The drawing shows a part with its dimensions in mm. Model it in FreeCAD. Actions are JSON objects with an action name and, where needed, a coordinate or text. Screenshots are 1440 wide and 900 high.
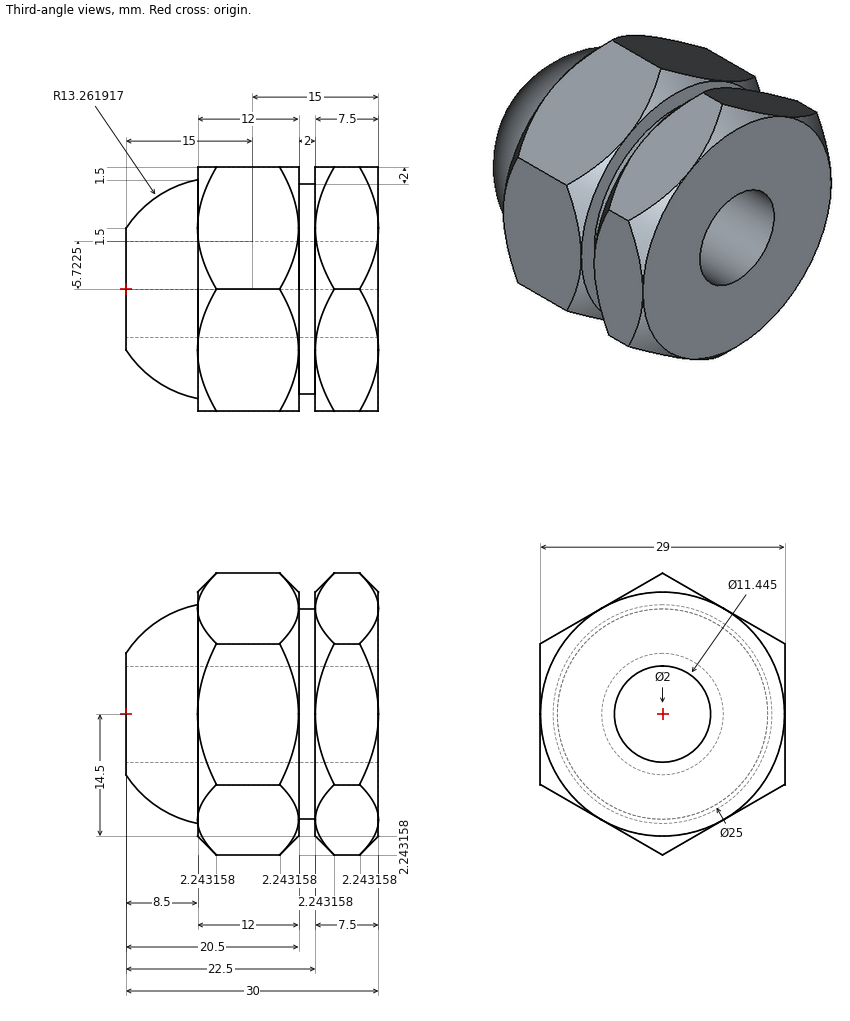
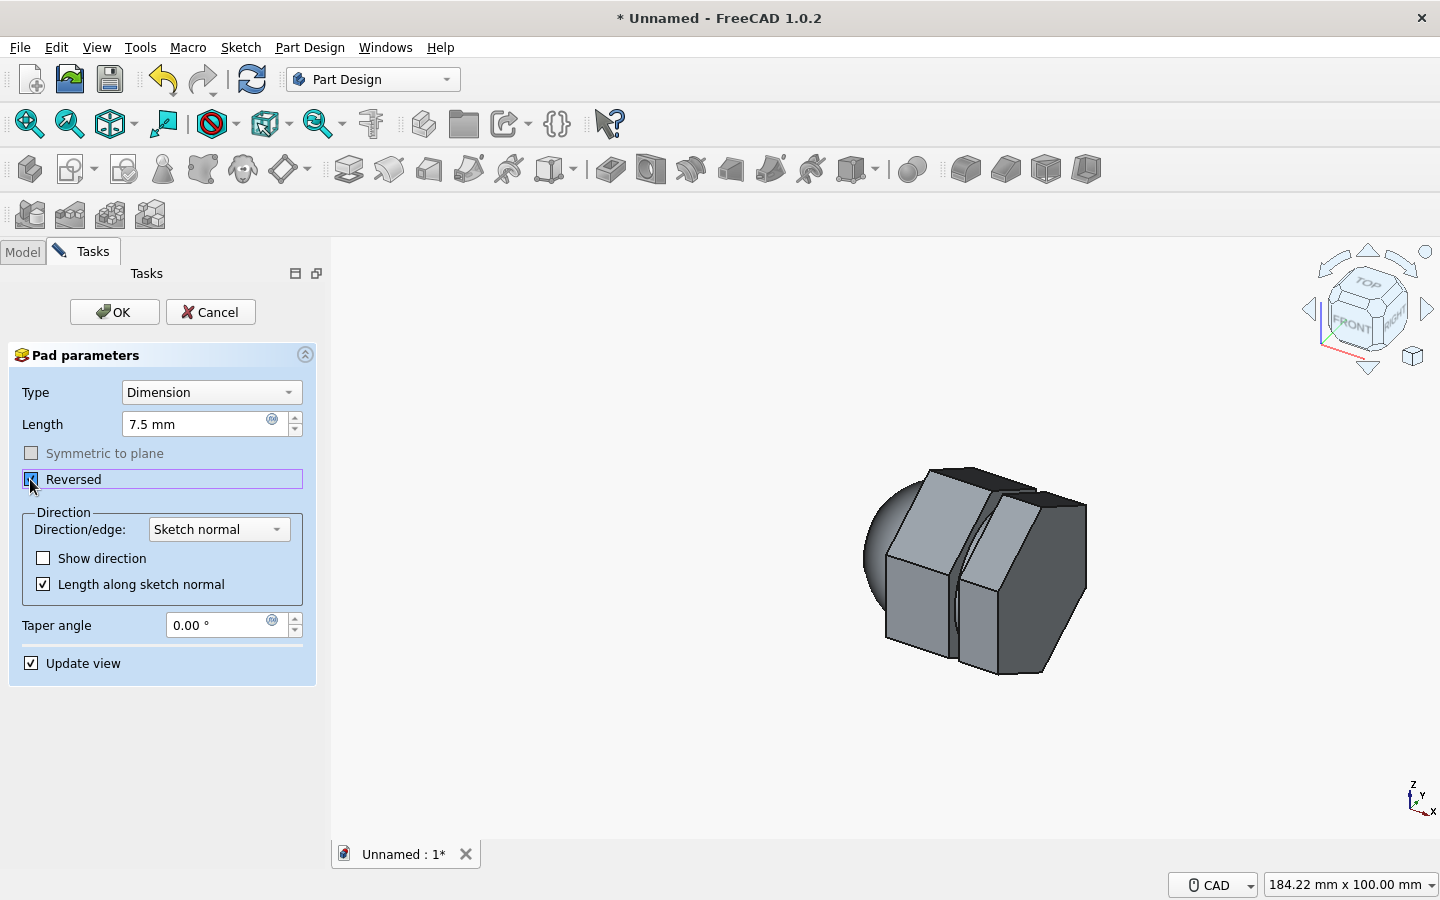
{"action": "left_click", "coordinate": [115, 312]}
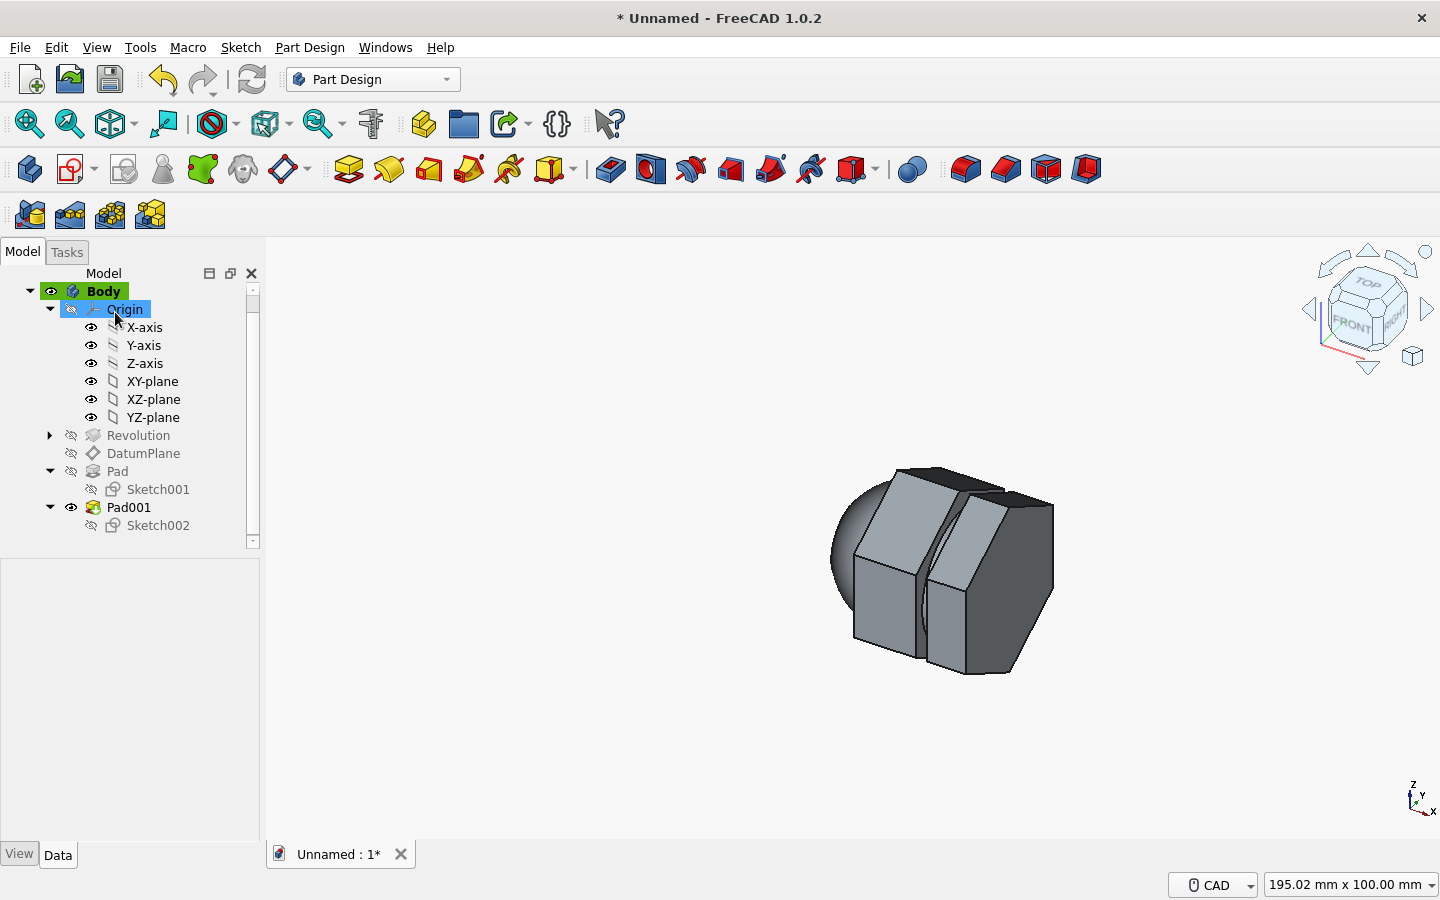
{"action": "left_click", "coordinate": [70, 170]}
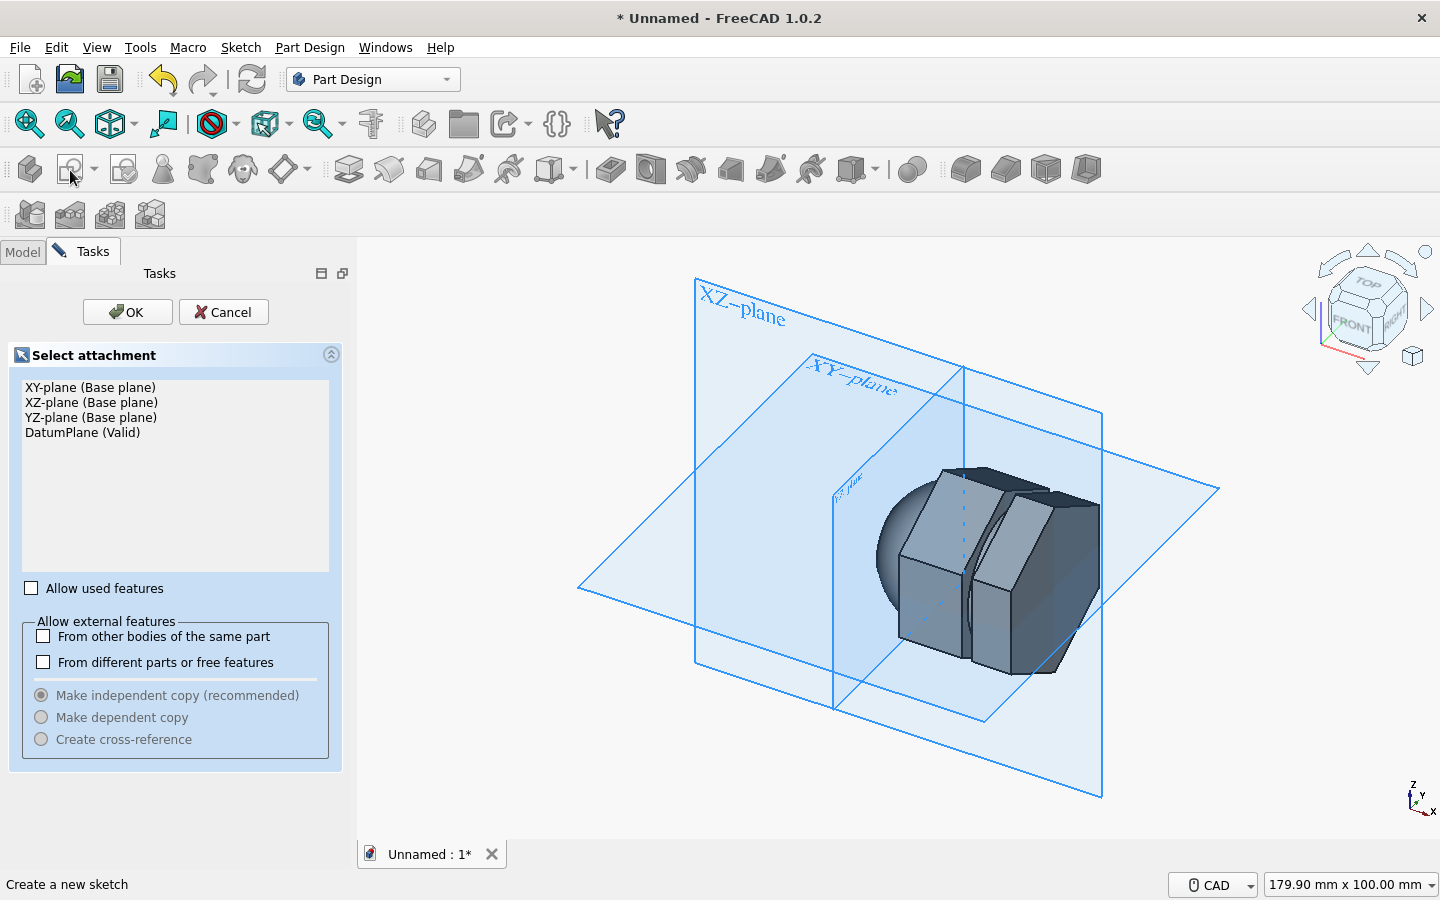
{"action": "left_click", "coordinate": [82, 402]}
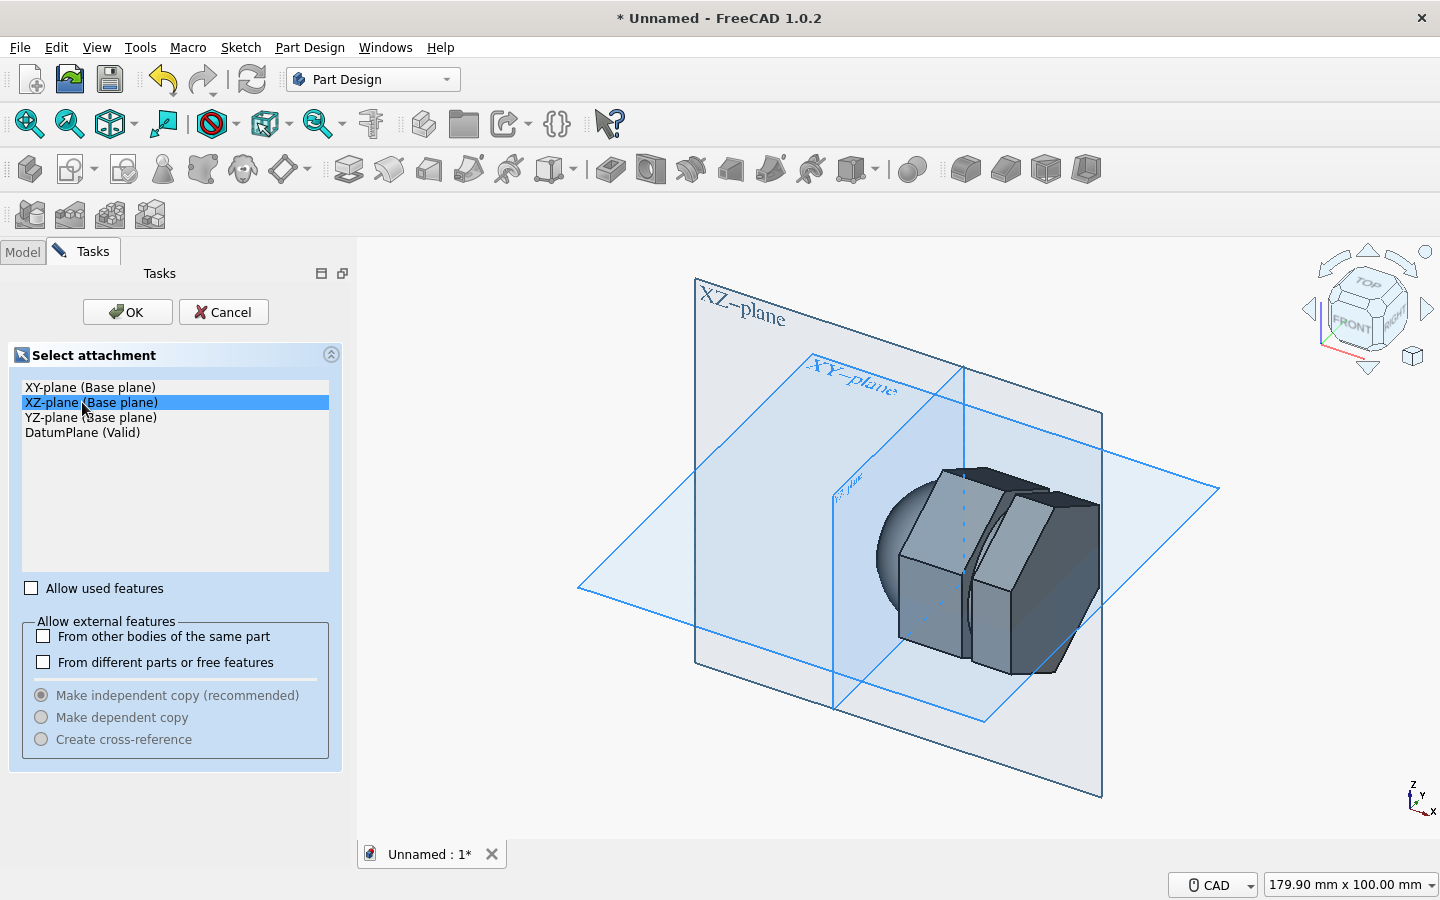
{"action": "left_click", "coordinate": [128, 312]}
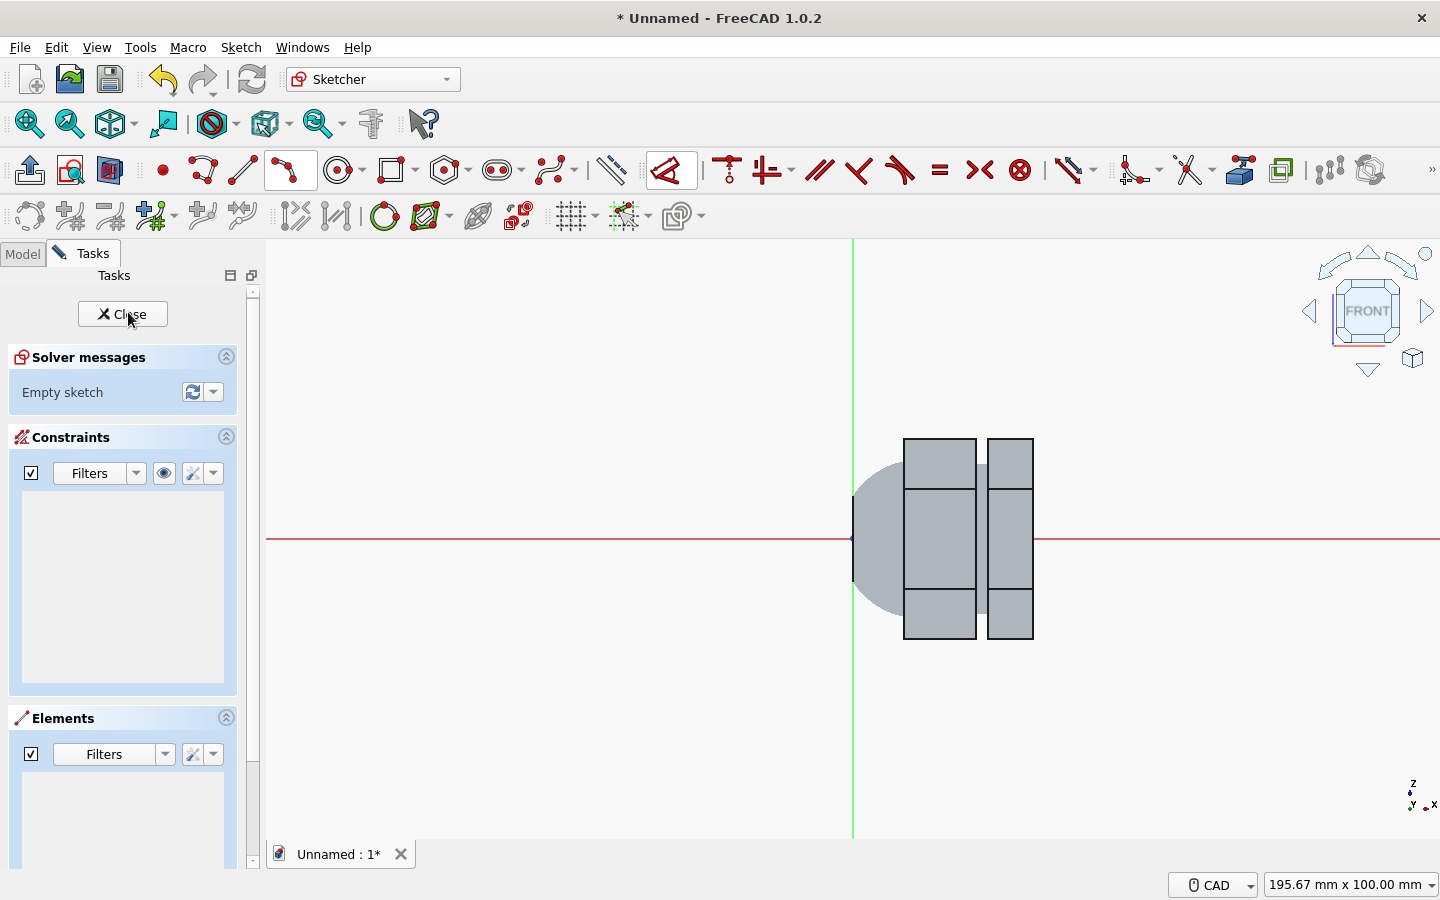
{"action": "key", "text": "q s"}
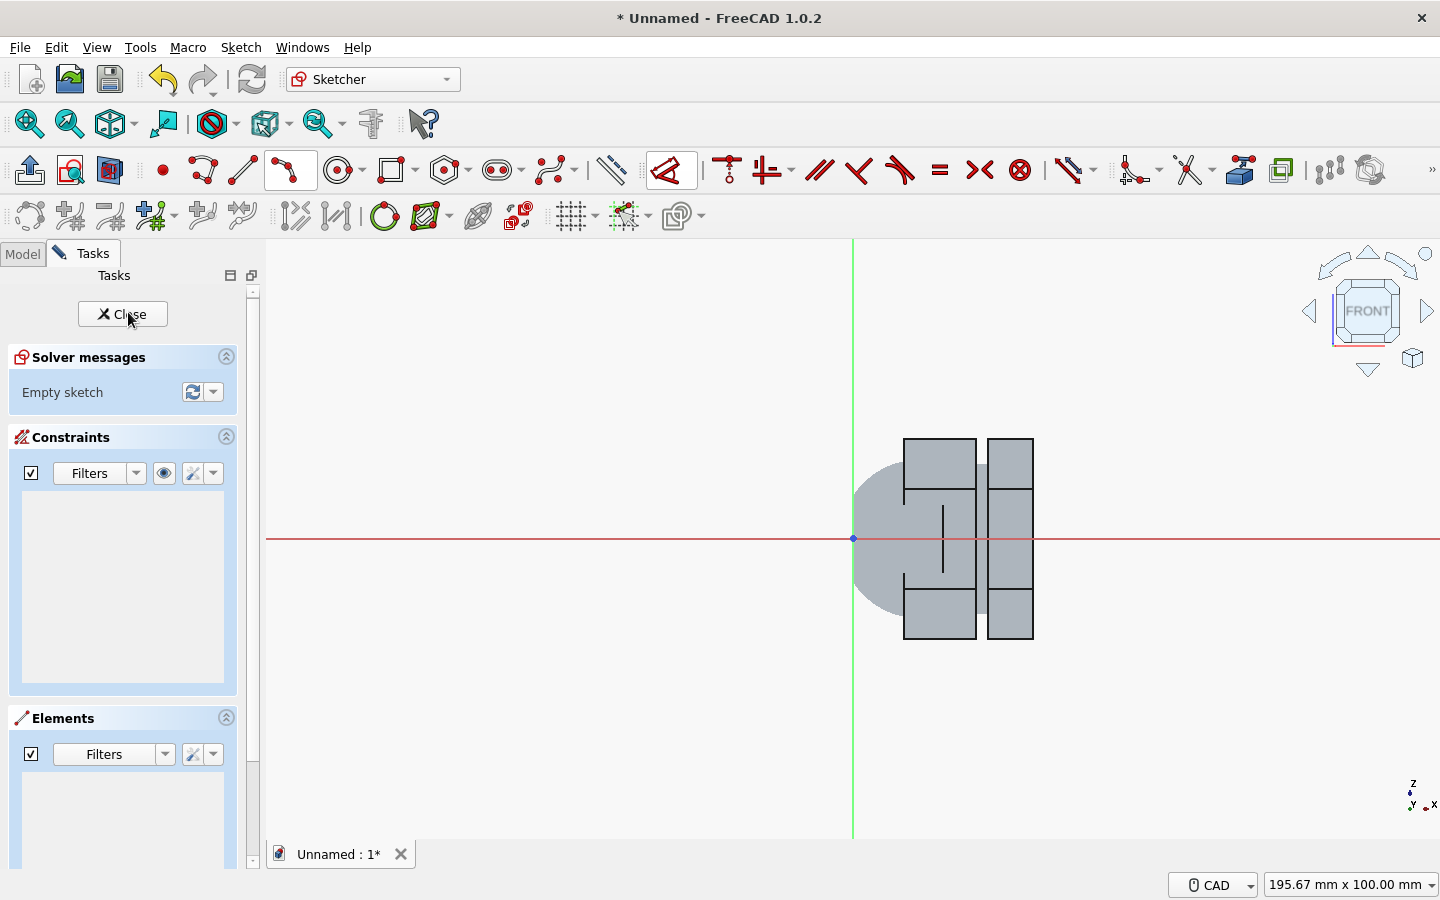
{"action": "scroll", "coordinate": [995, 606], "scroll_direction": "up", "scroll_amount": 7}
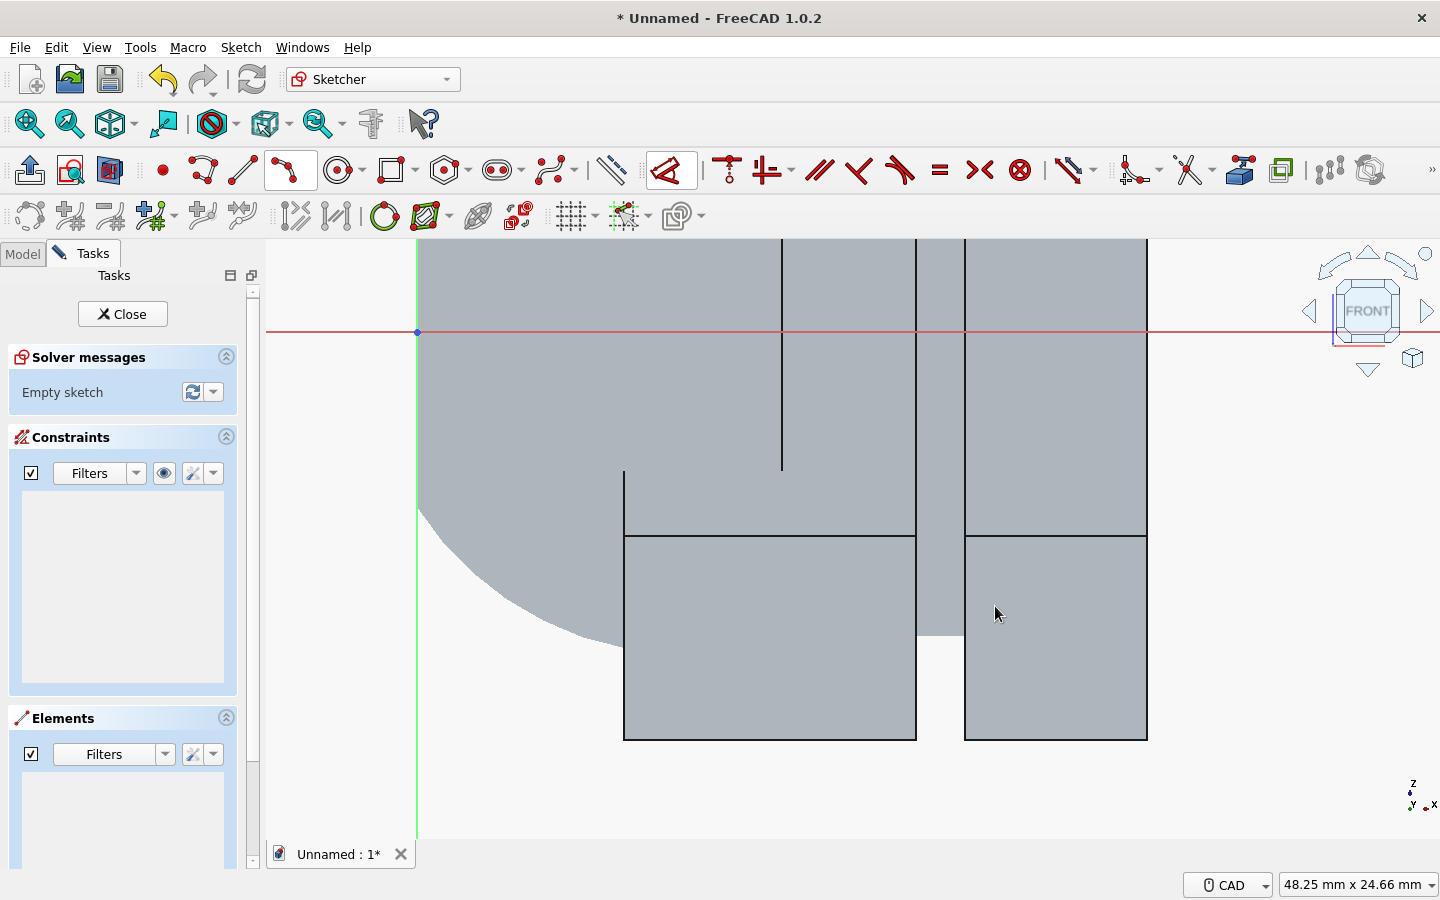
{"action": "left_click", "coordinate": [204, 170]}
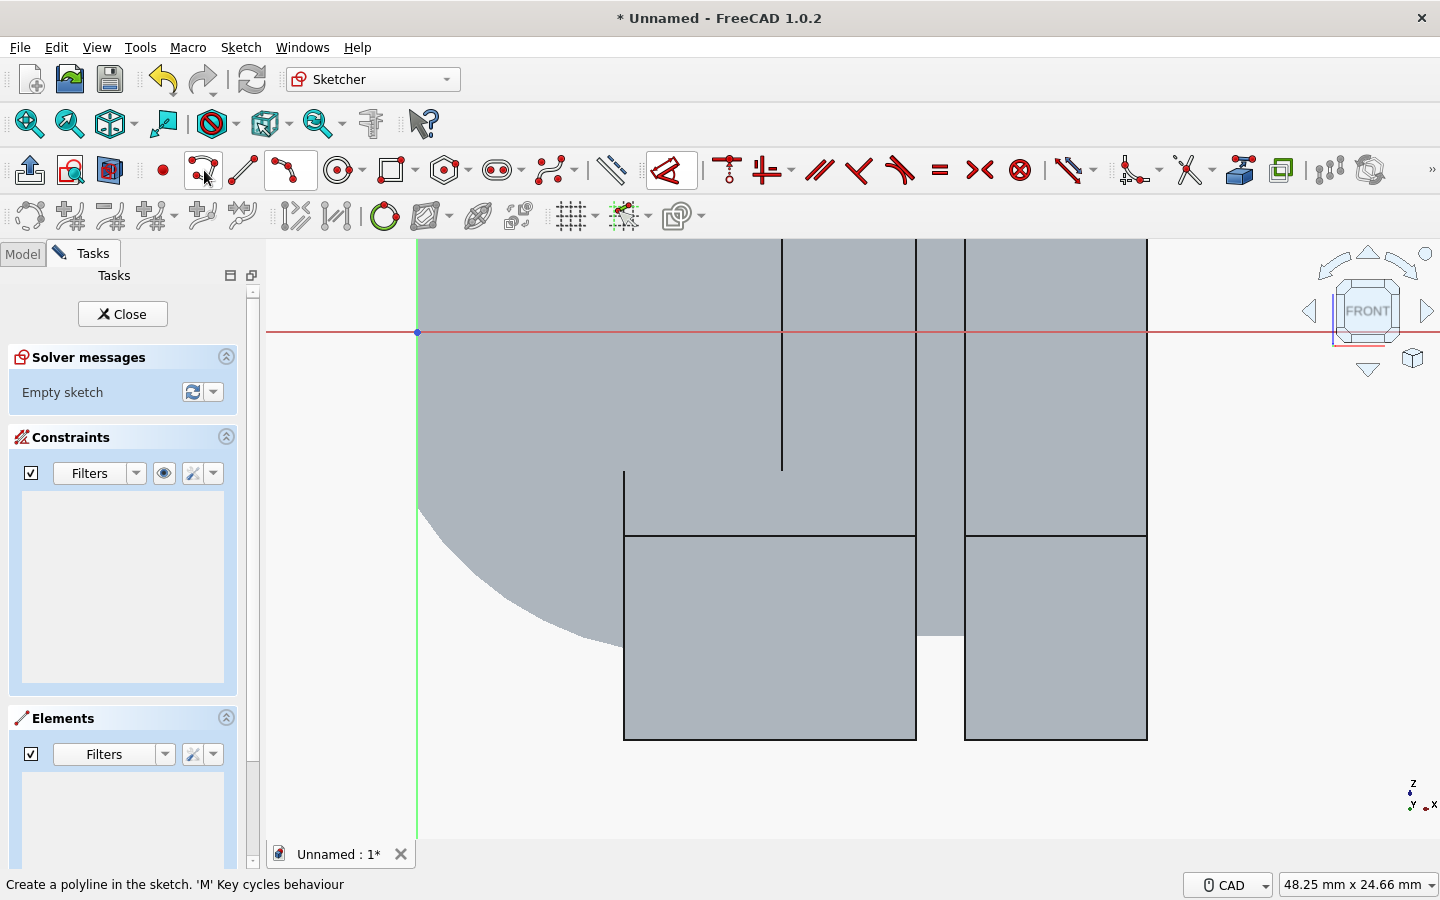
{"action": "left_click", "coordinate": [861, 740]}
{"action": "left_click", "coordinate": [916, 685]}
{"action": "left_click", "coordinate": [916, 740]}
{"action": "left_click", "coordinate": [861, 741]}